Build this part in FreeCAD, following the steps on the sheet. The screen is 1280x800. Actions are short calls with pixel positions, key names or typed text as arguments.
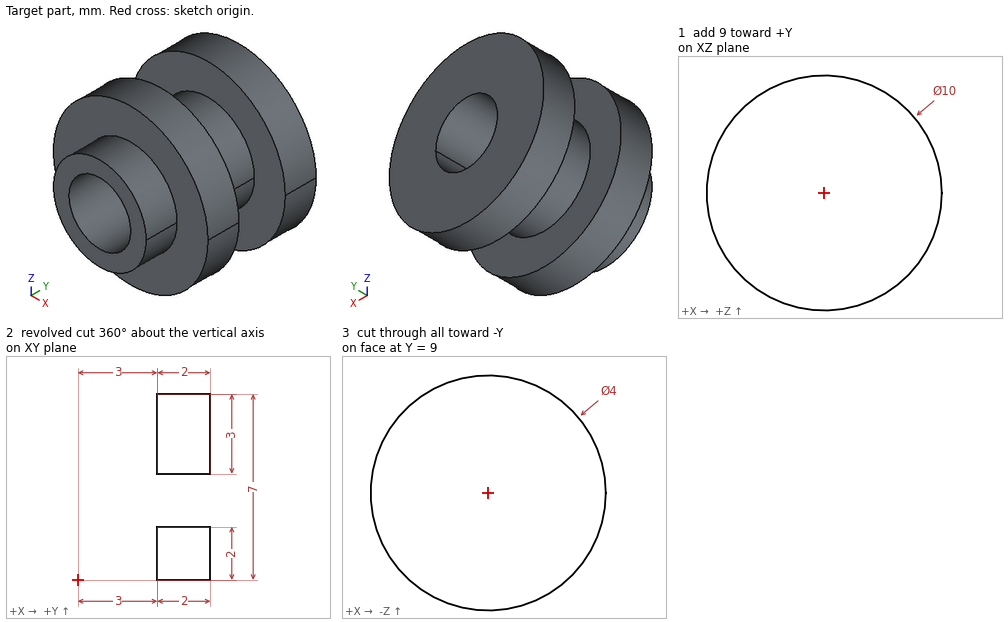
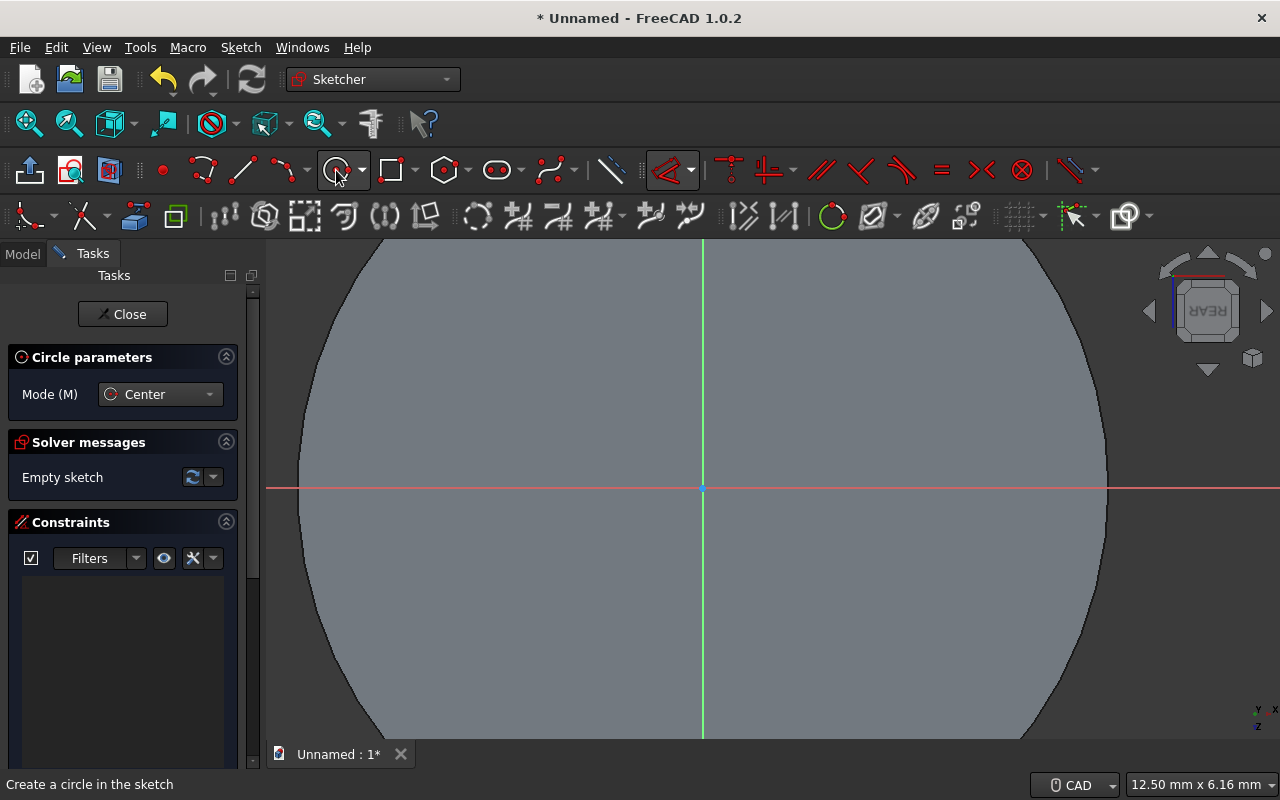
click(703, 488)
move(818, 373)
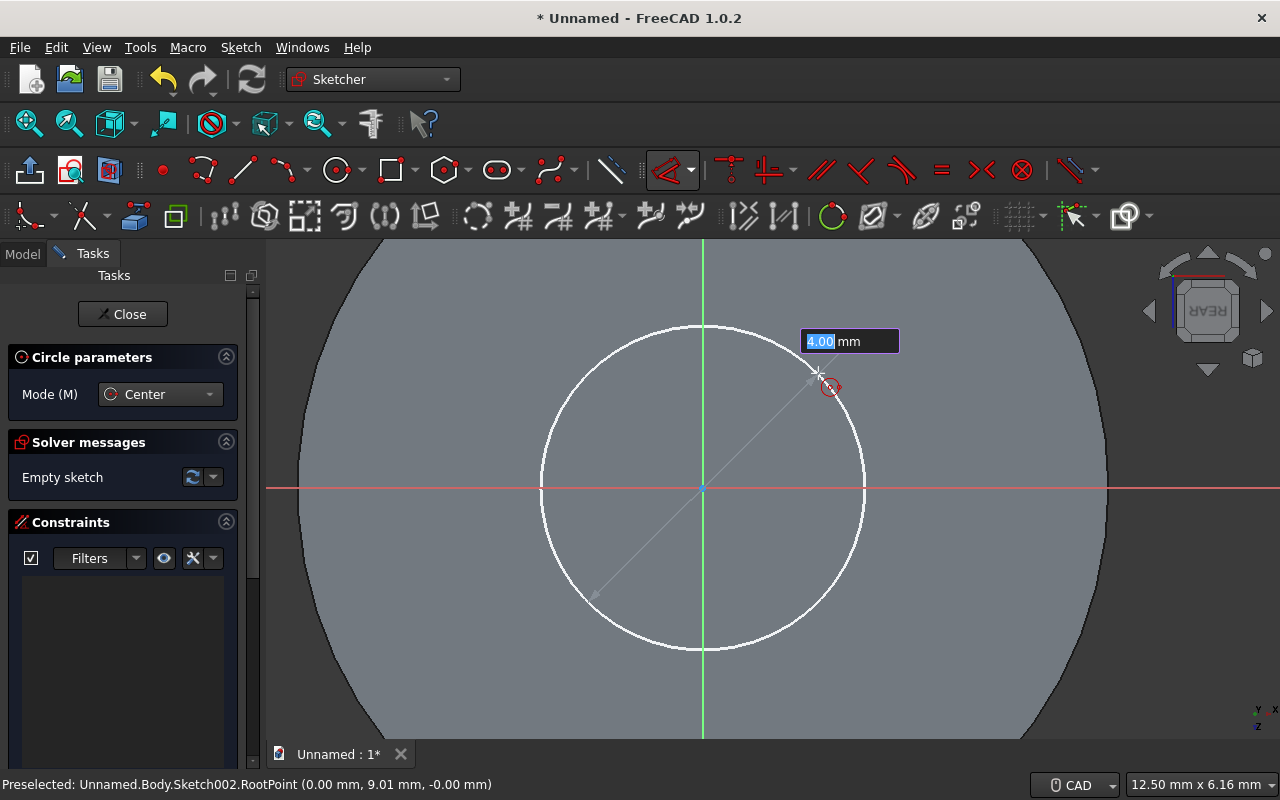
text(4)
key(Return)
key(Escape)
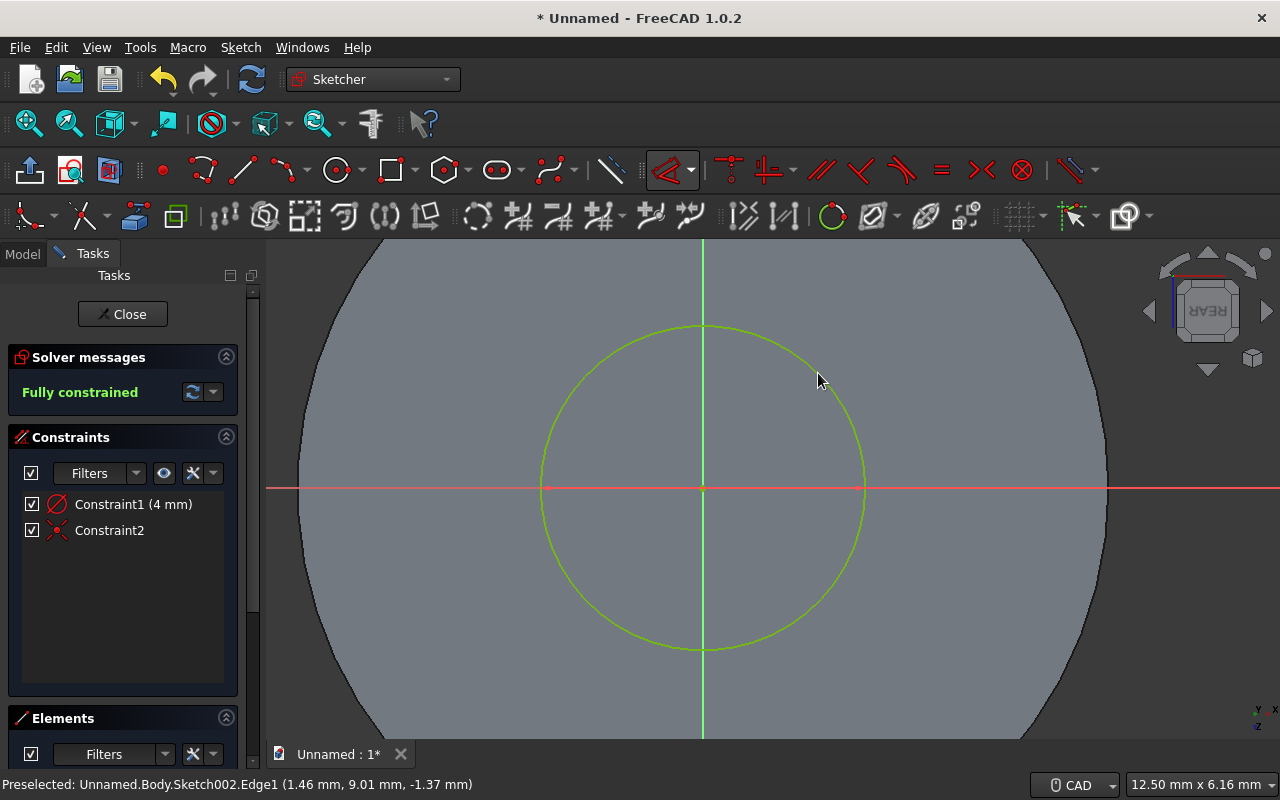
click(123, 314)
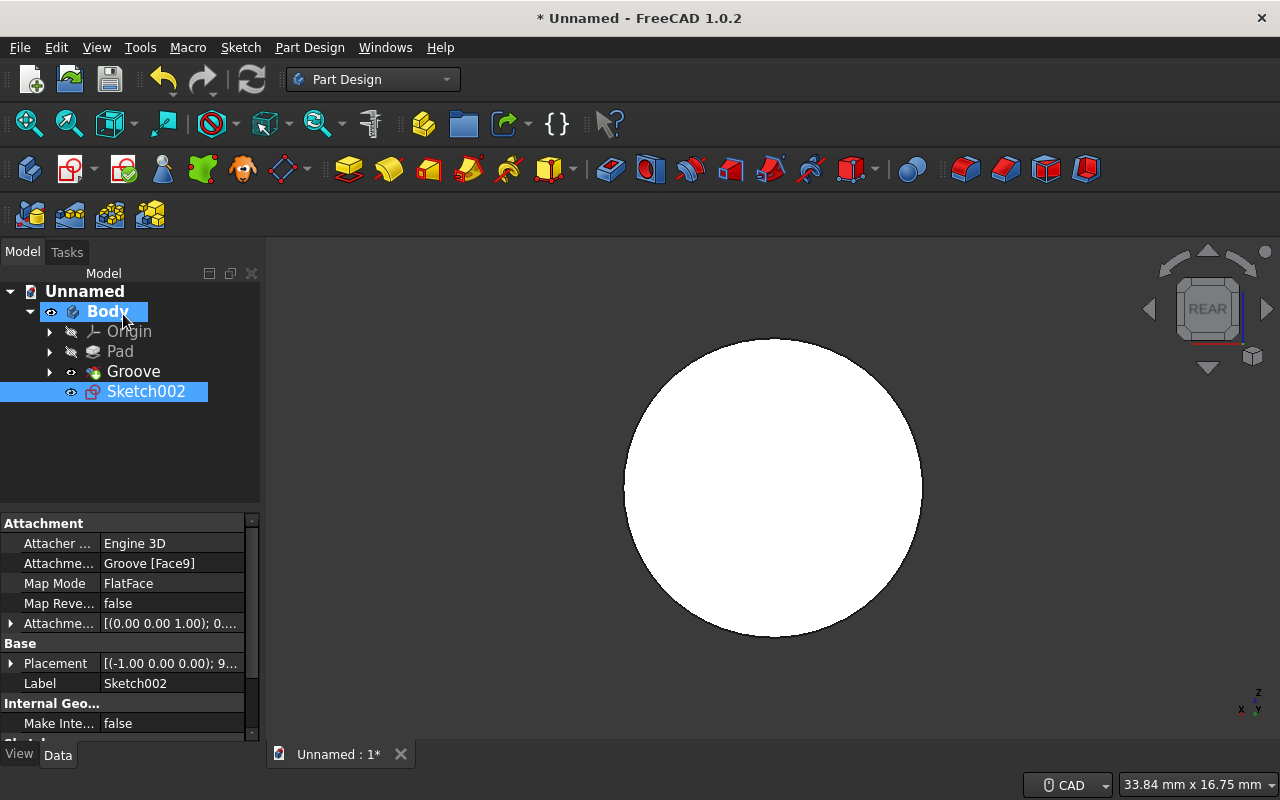
click(612, 170)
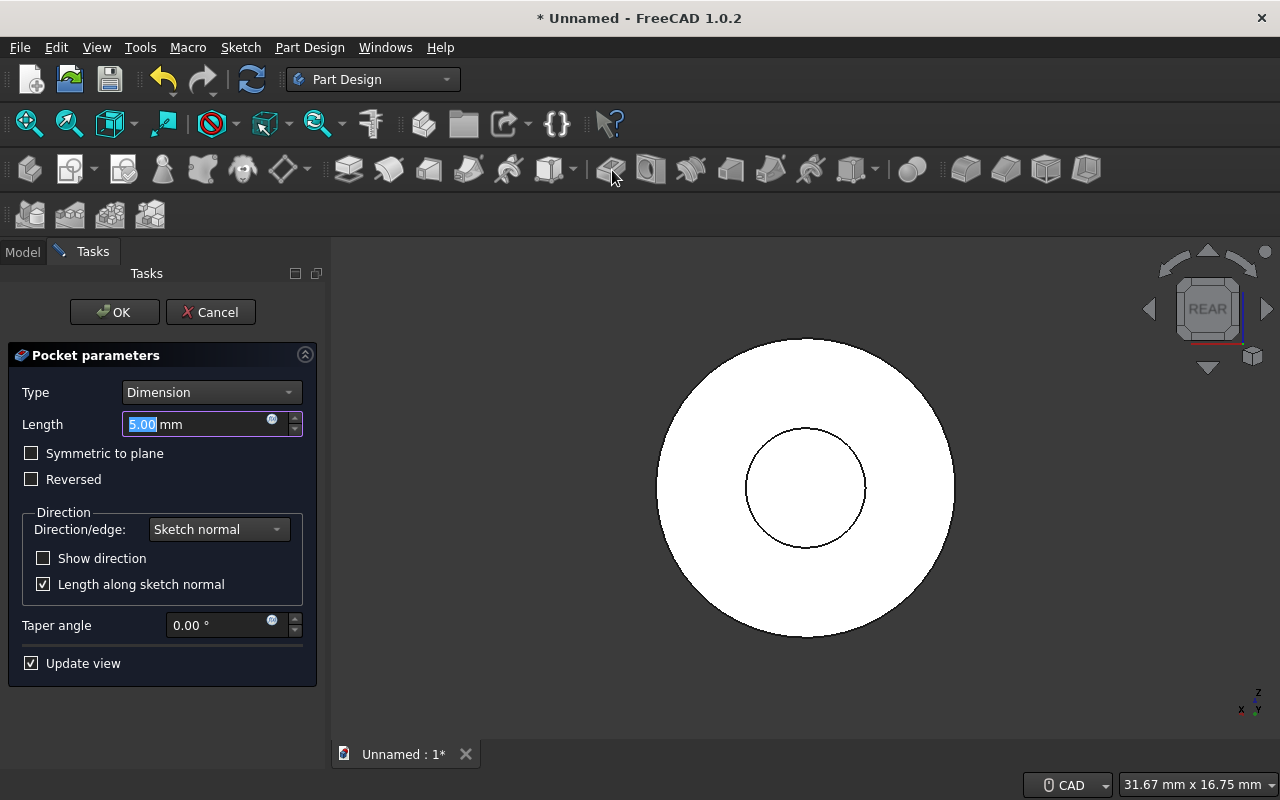
click(212, 392)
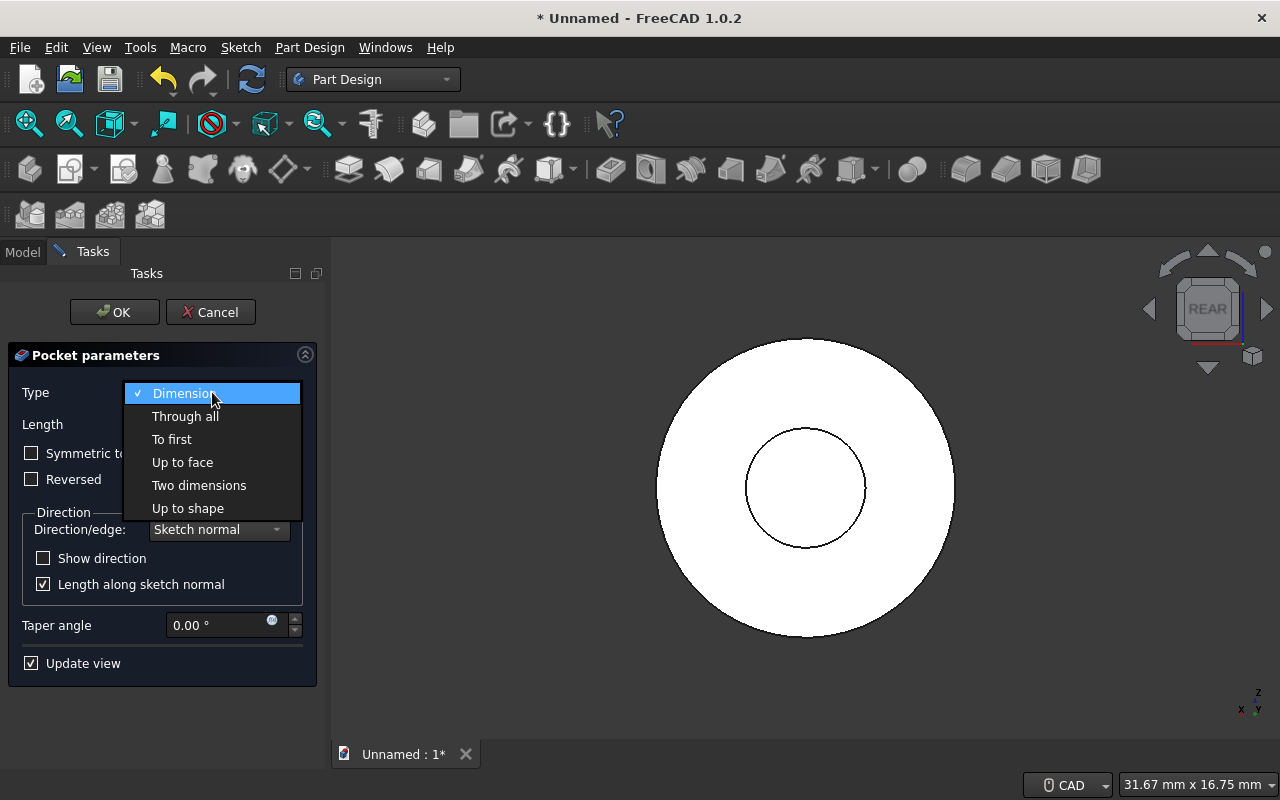
click(212, 416)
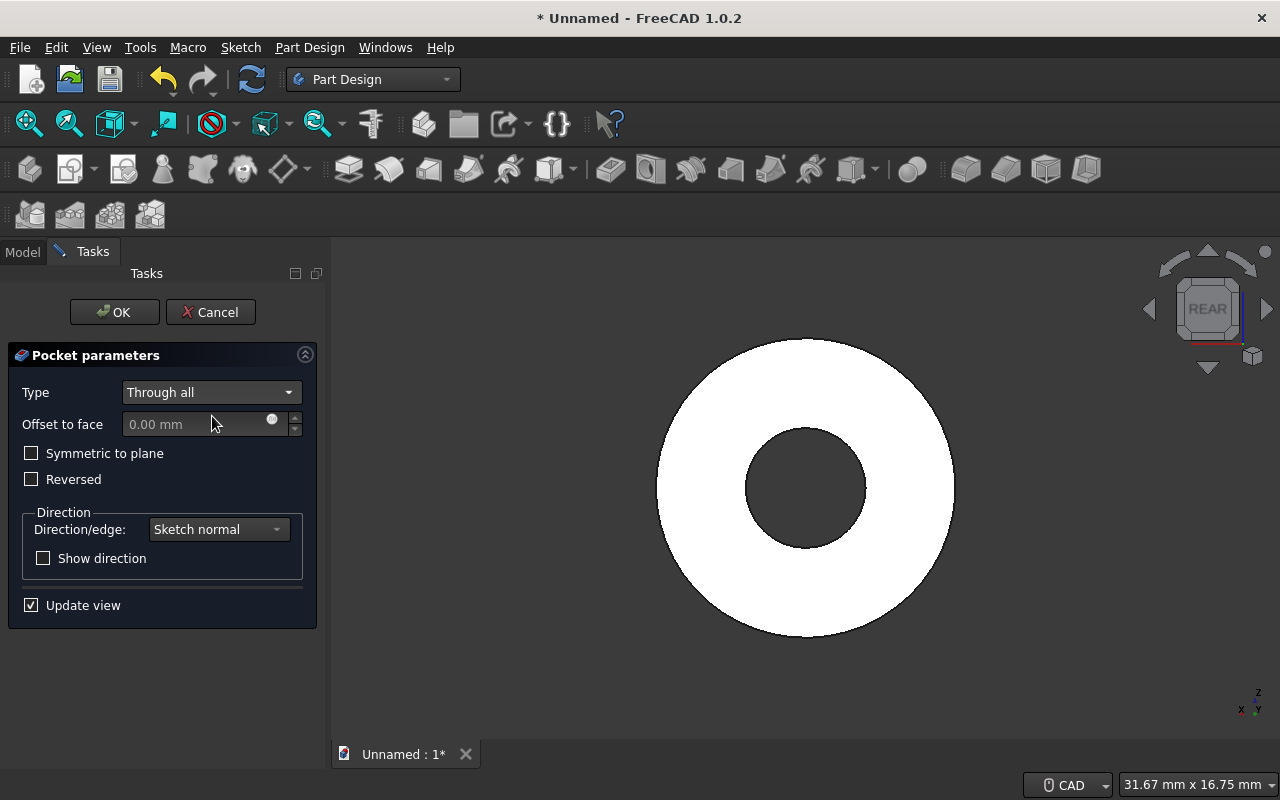
click(115, 312)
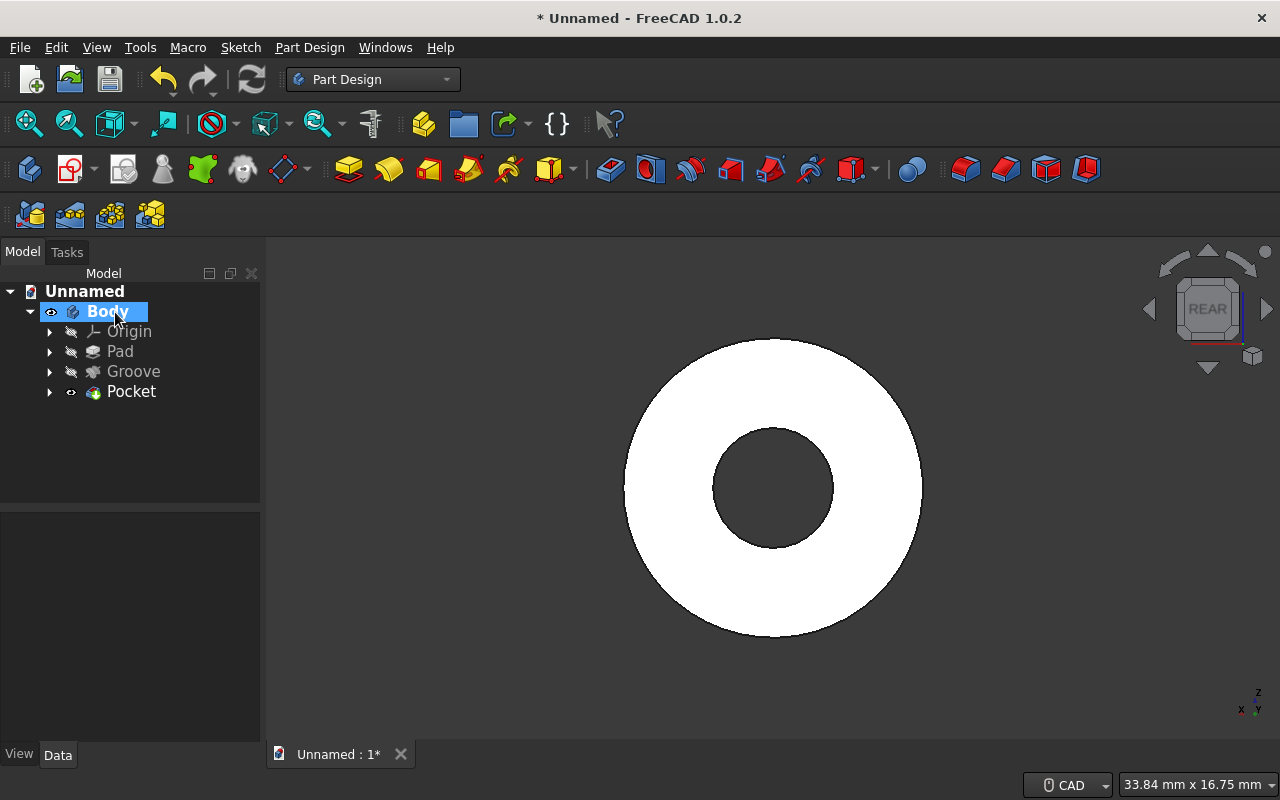
key(0)